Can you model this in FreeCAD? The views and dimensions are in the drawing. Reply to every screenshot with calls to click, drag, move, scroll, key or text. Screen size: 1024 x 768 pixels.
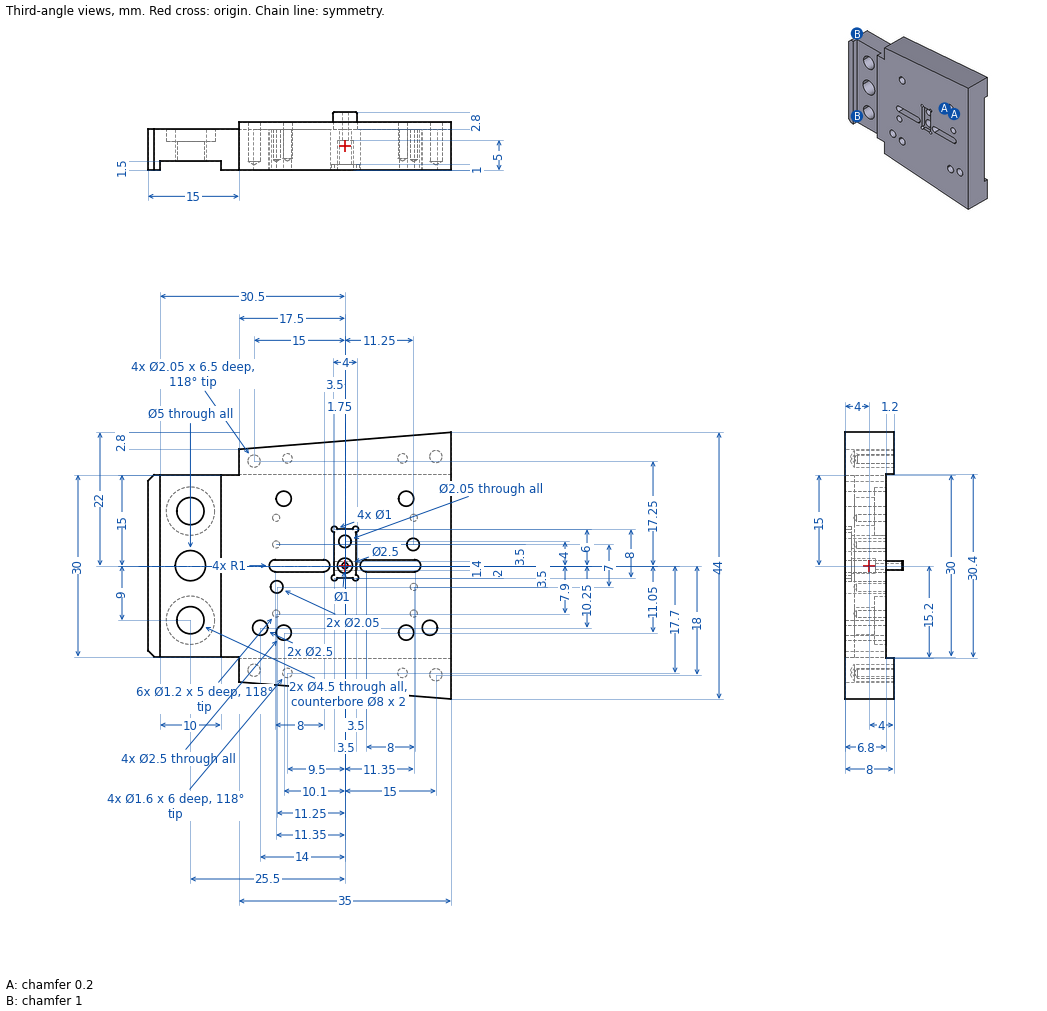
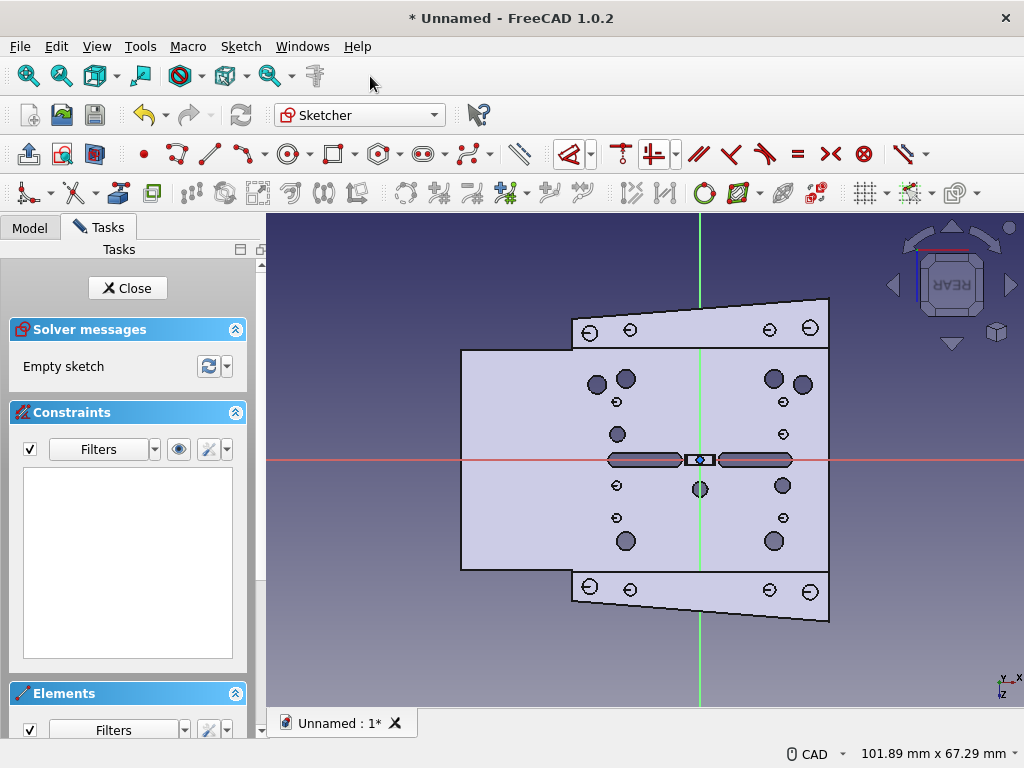
scroll(625, 460, up, 3)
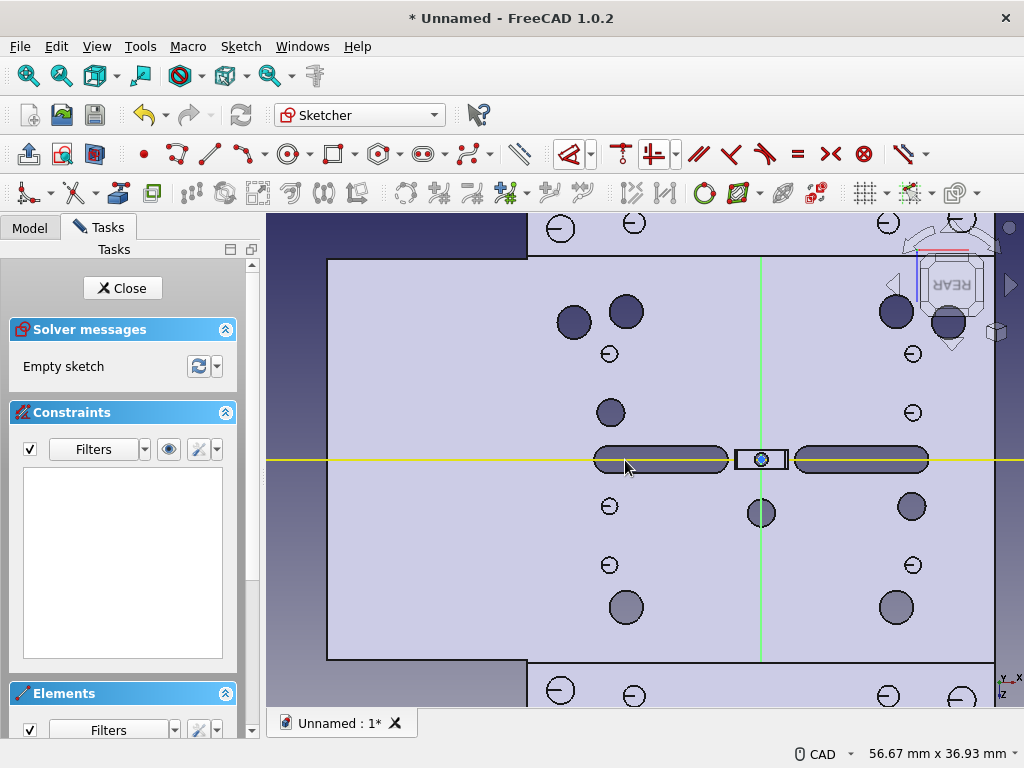
click(288, 154)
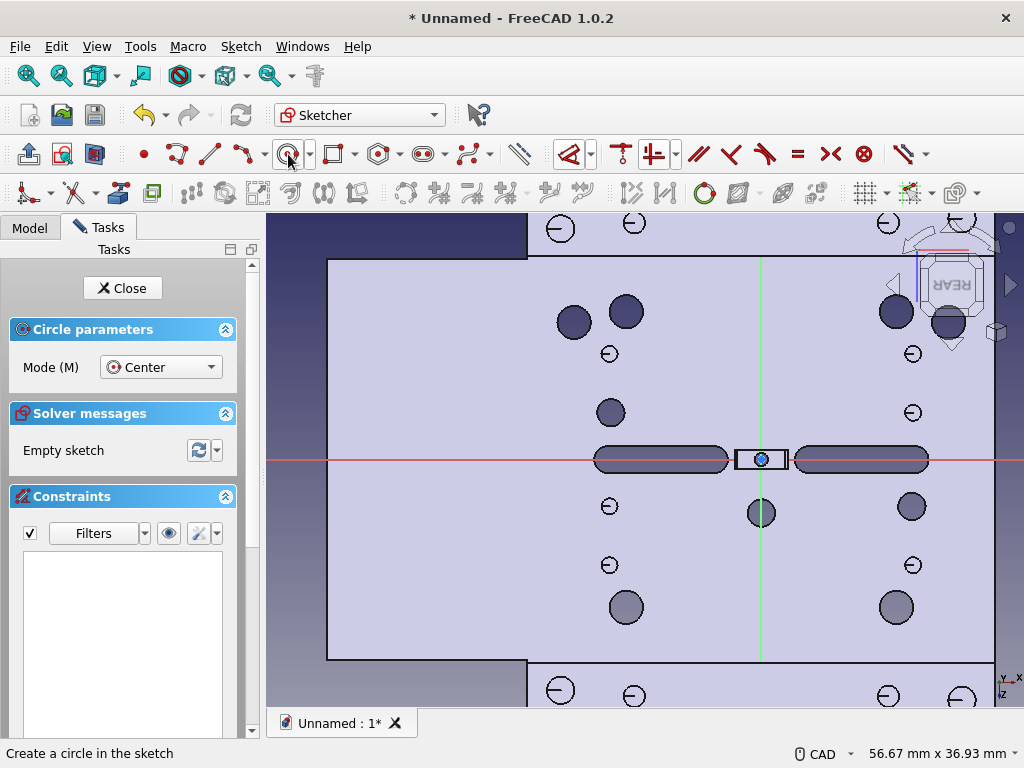
click(420, 339)
move(442, 318)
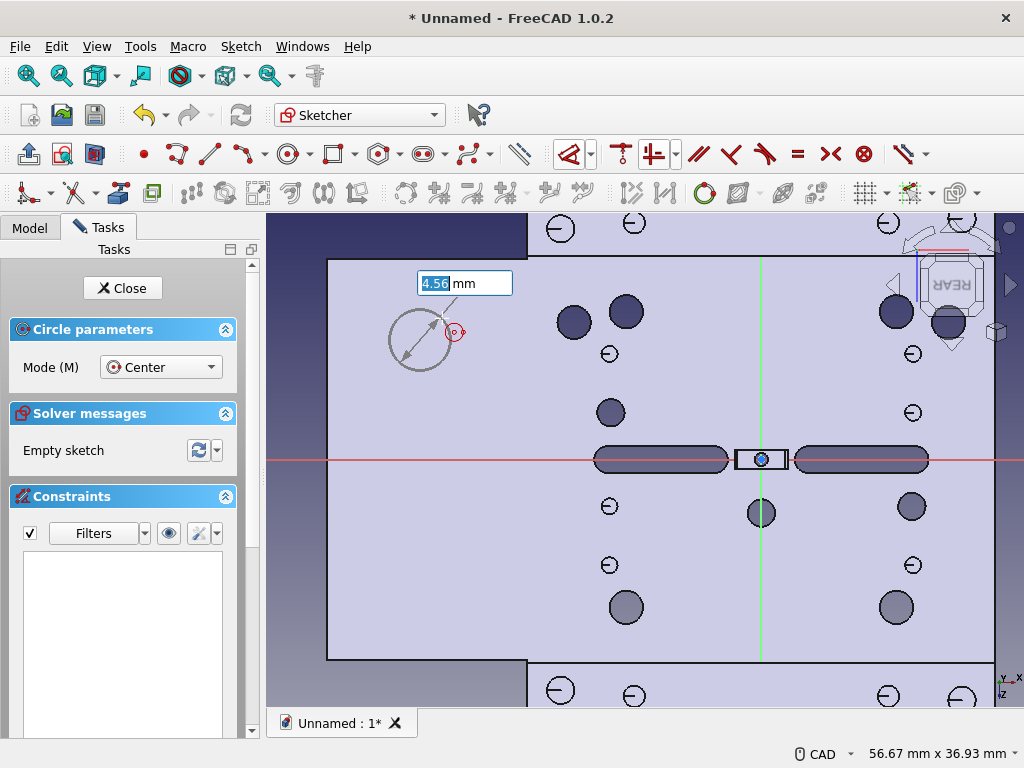
text(4.5)
key(Return)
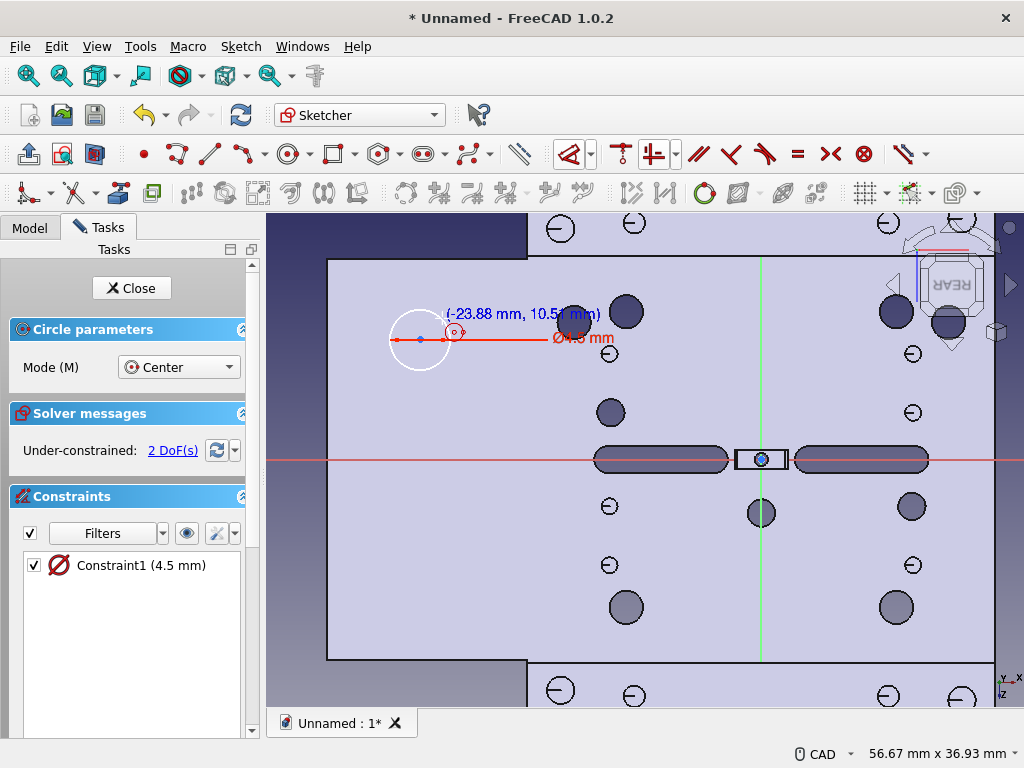
click(420, 580)
move(442, 559)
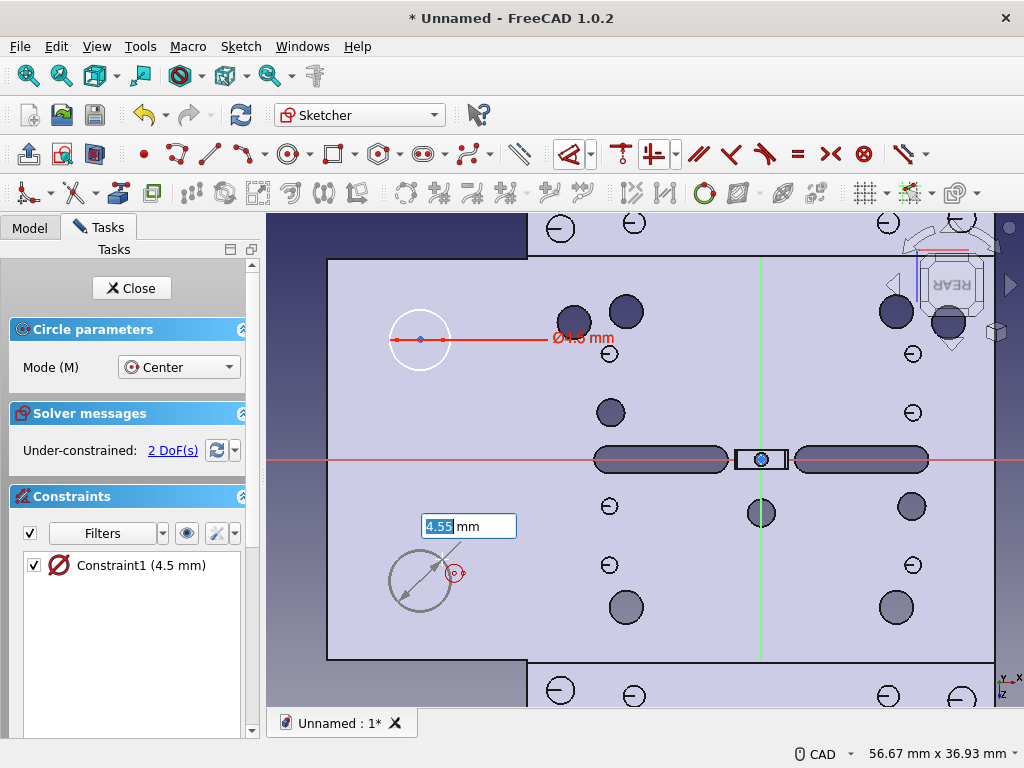
text(4.5)
key(Return)
key(Escape)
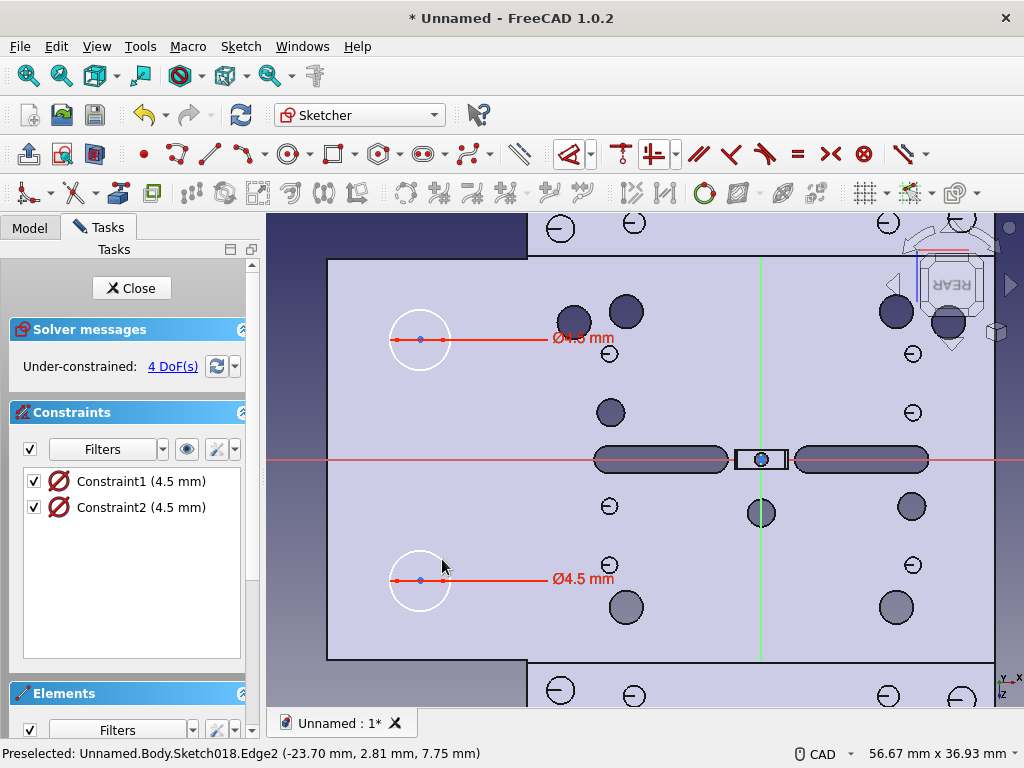
click(420, 340)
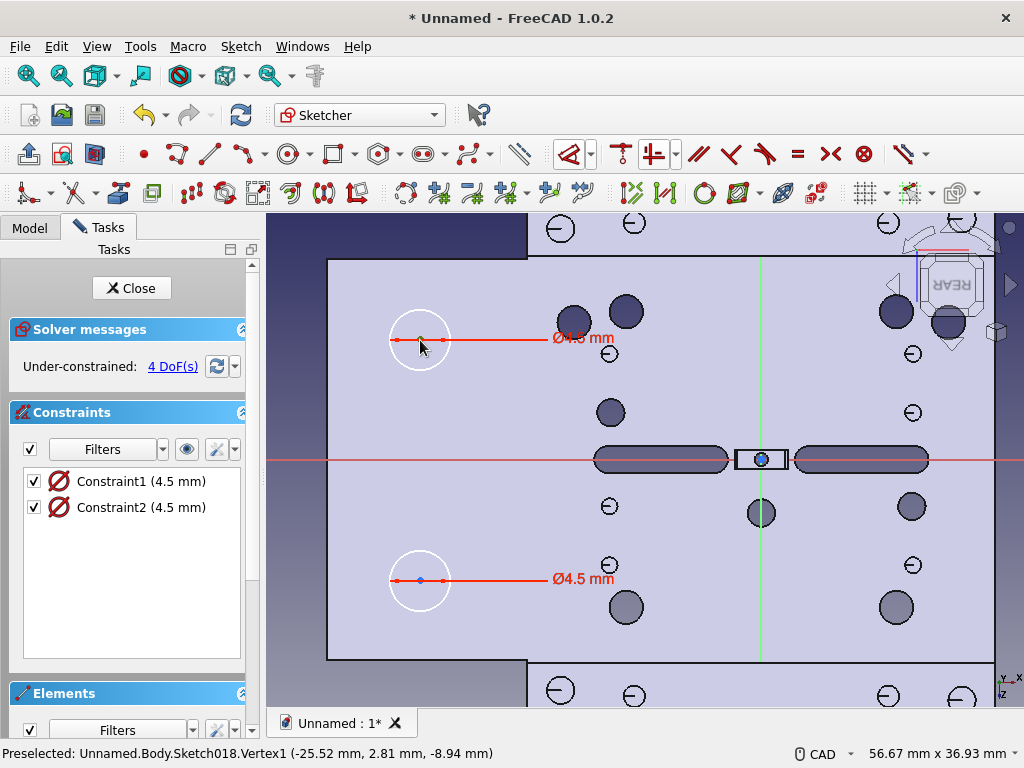
click(420, 581)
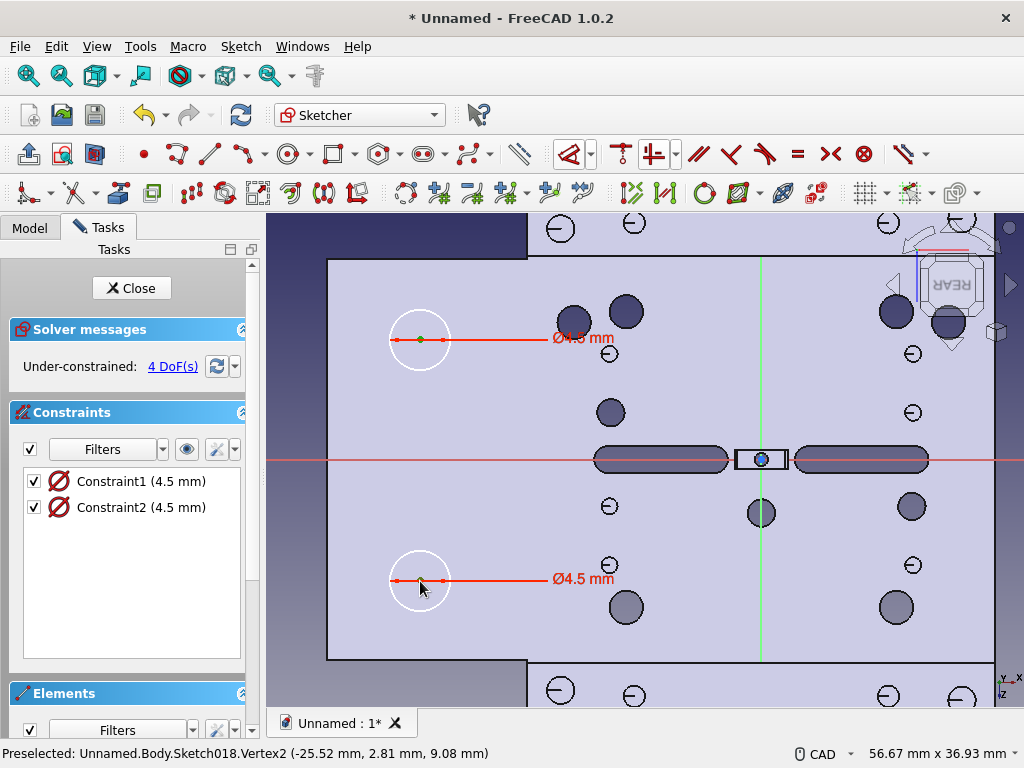
click(334, 460)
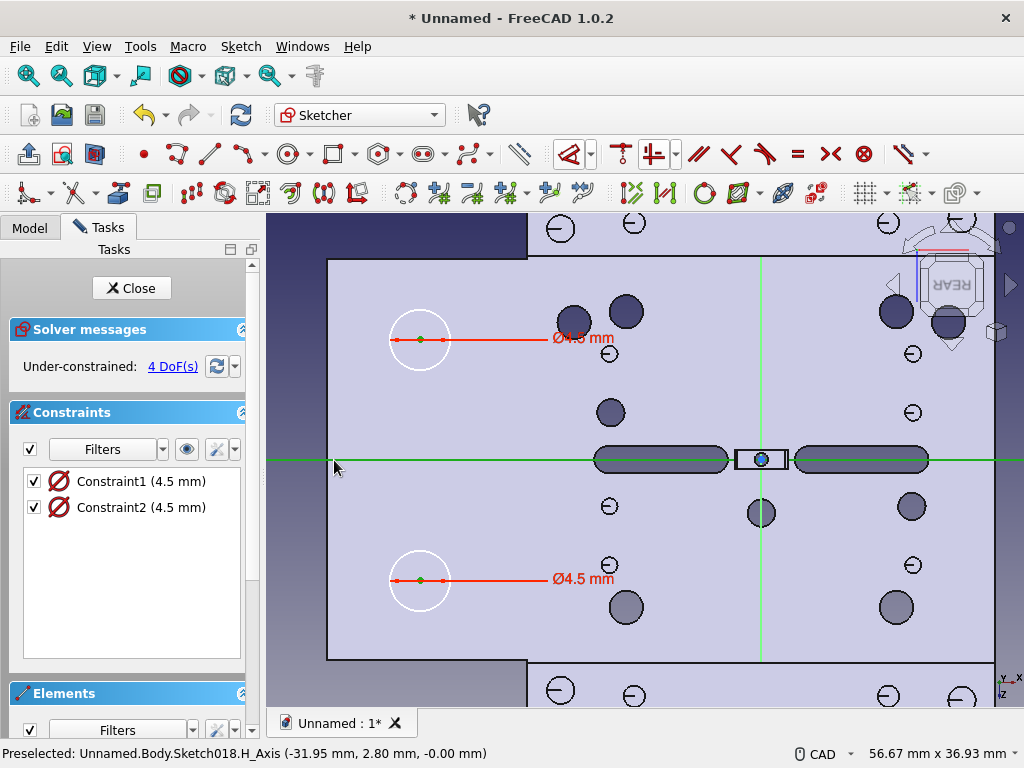
click(831, 154)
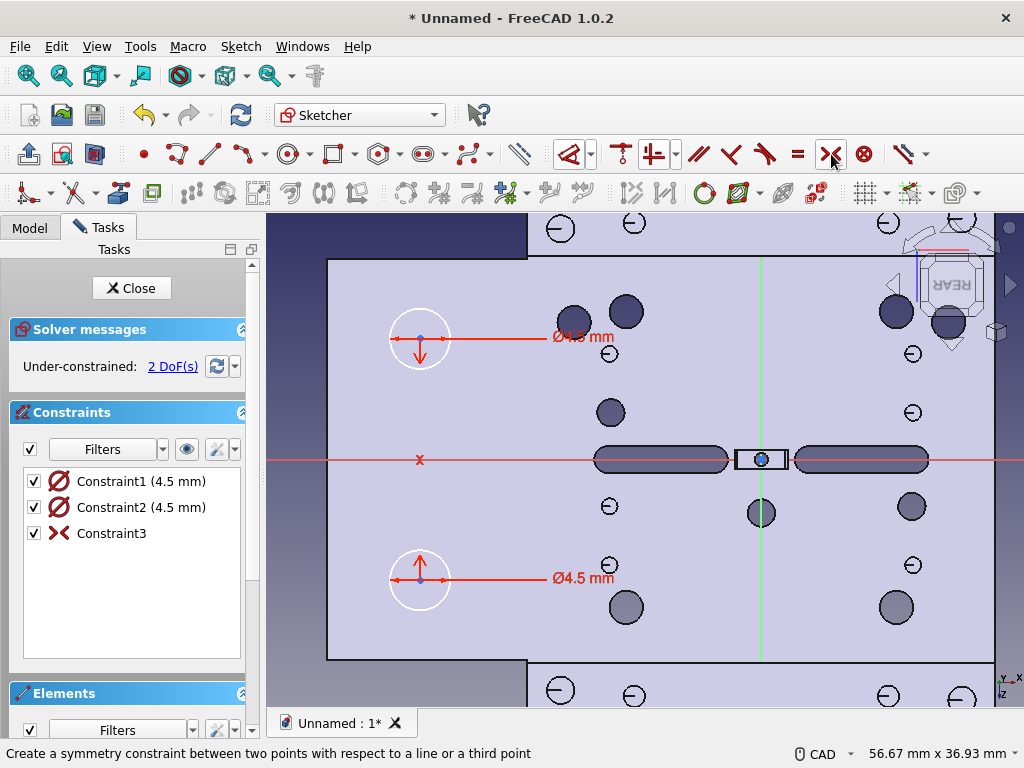
click(420, 339)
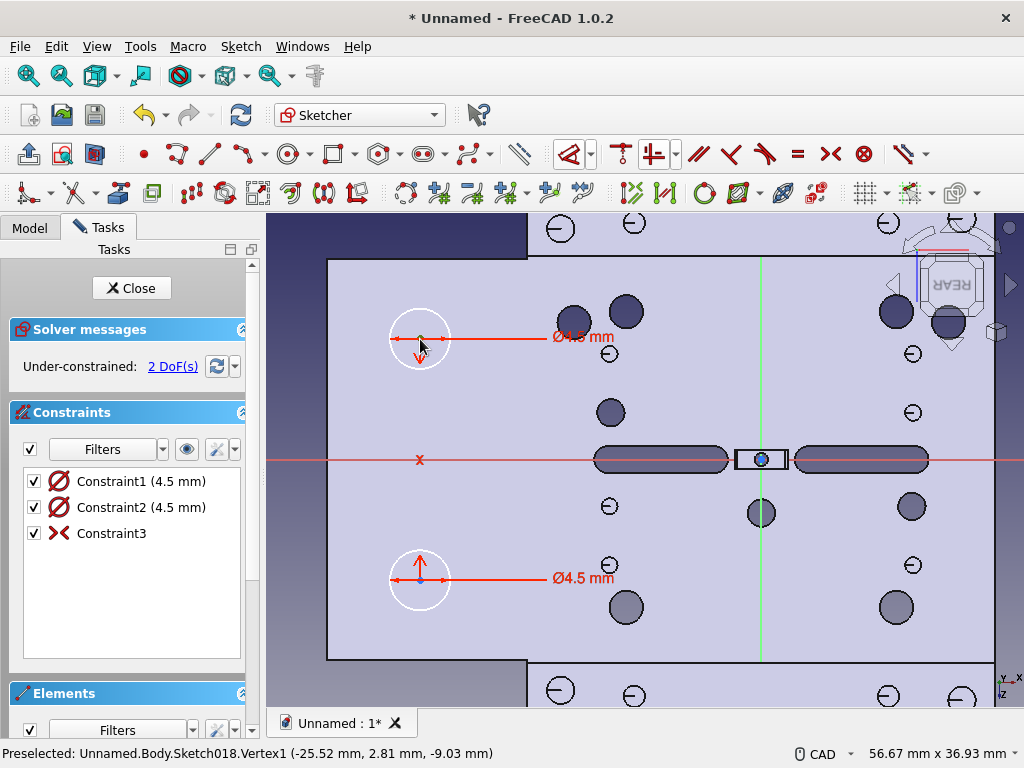
key(i)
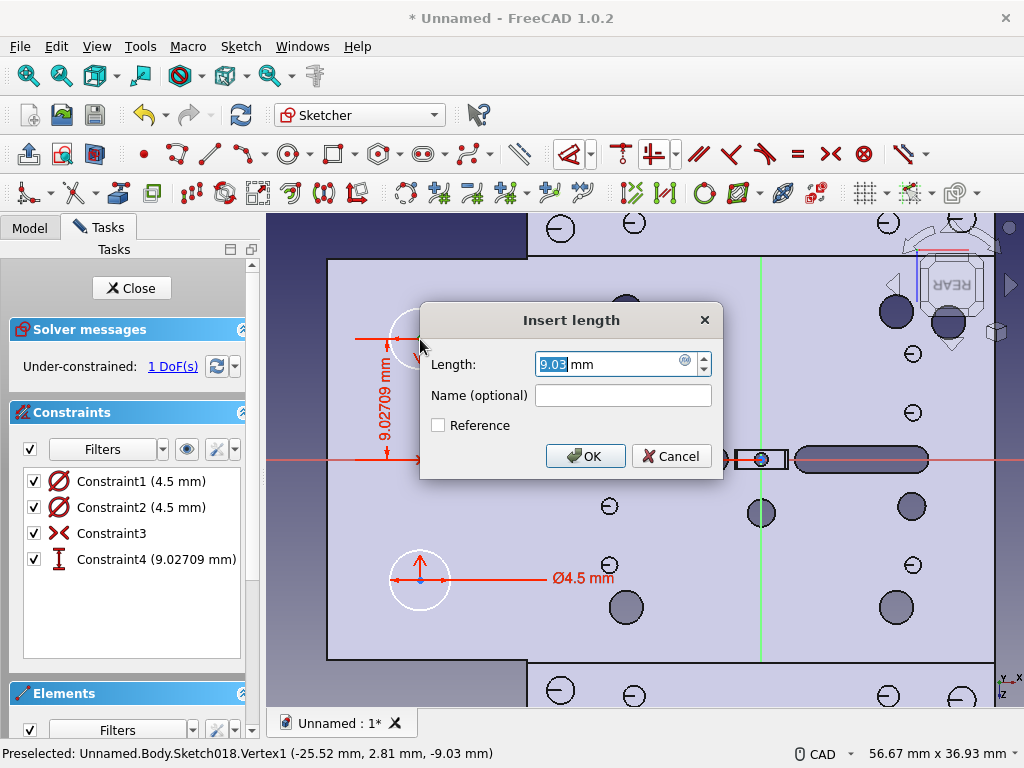
text(9)
key(Return)